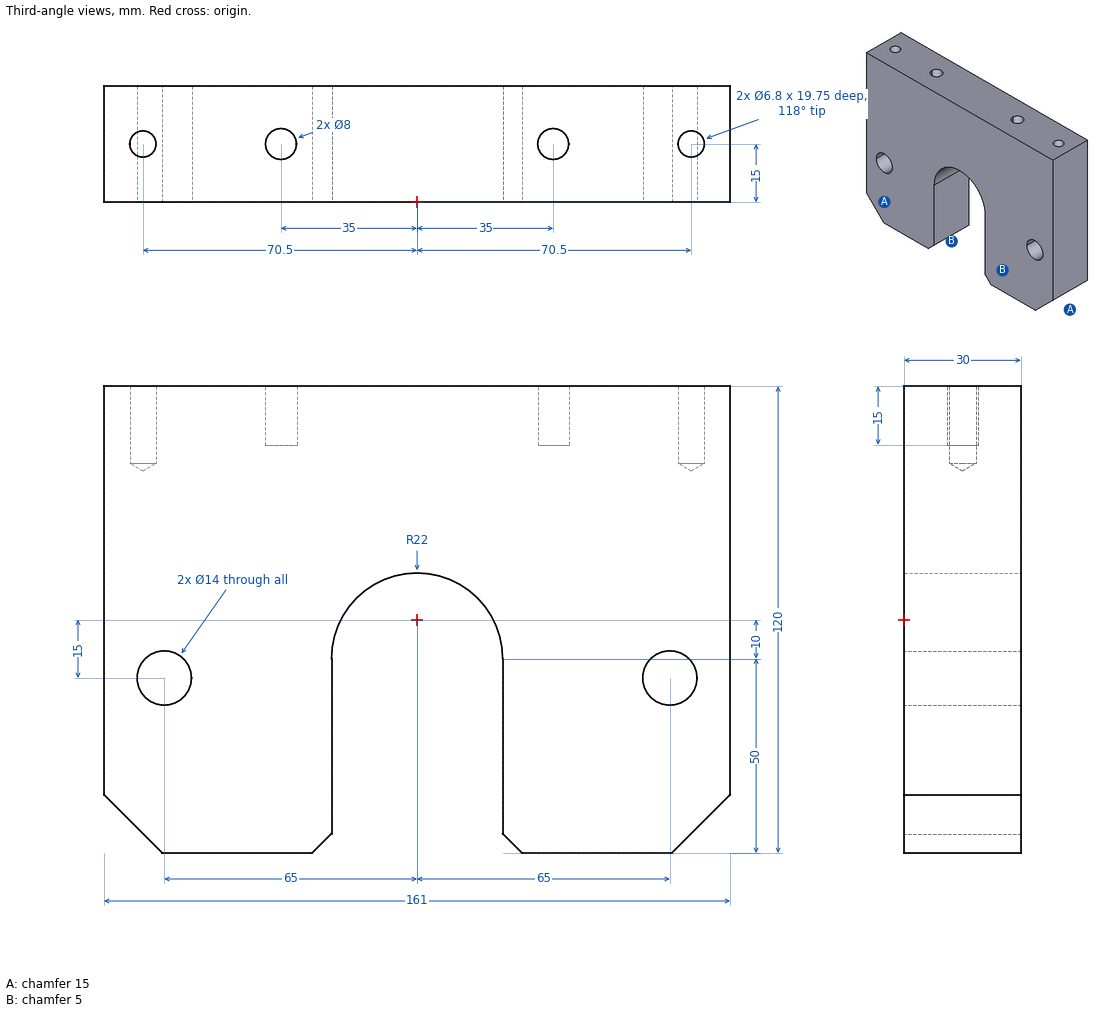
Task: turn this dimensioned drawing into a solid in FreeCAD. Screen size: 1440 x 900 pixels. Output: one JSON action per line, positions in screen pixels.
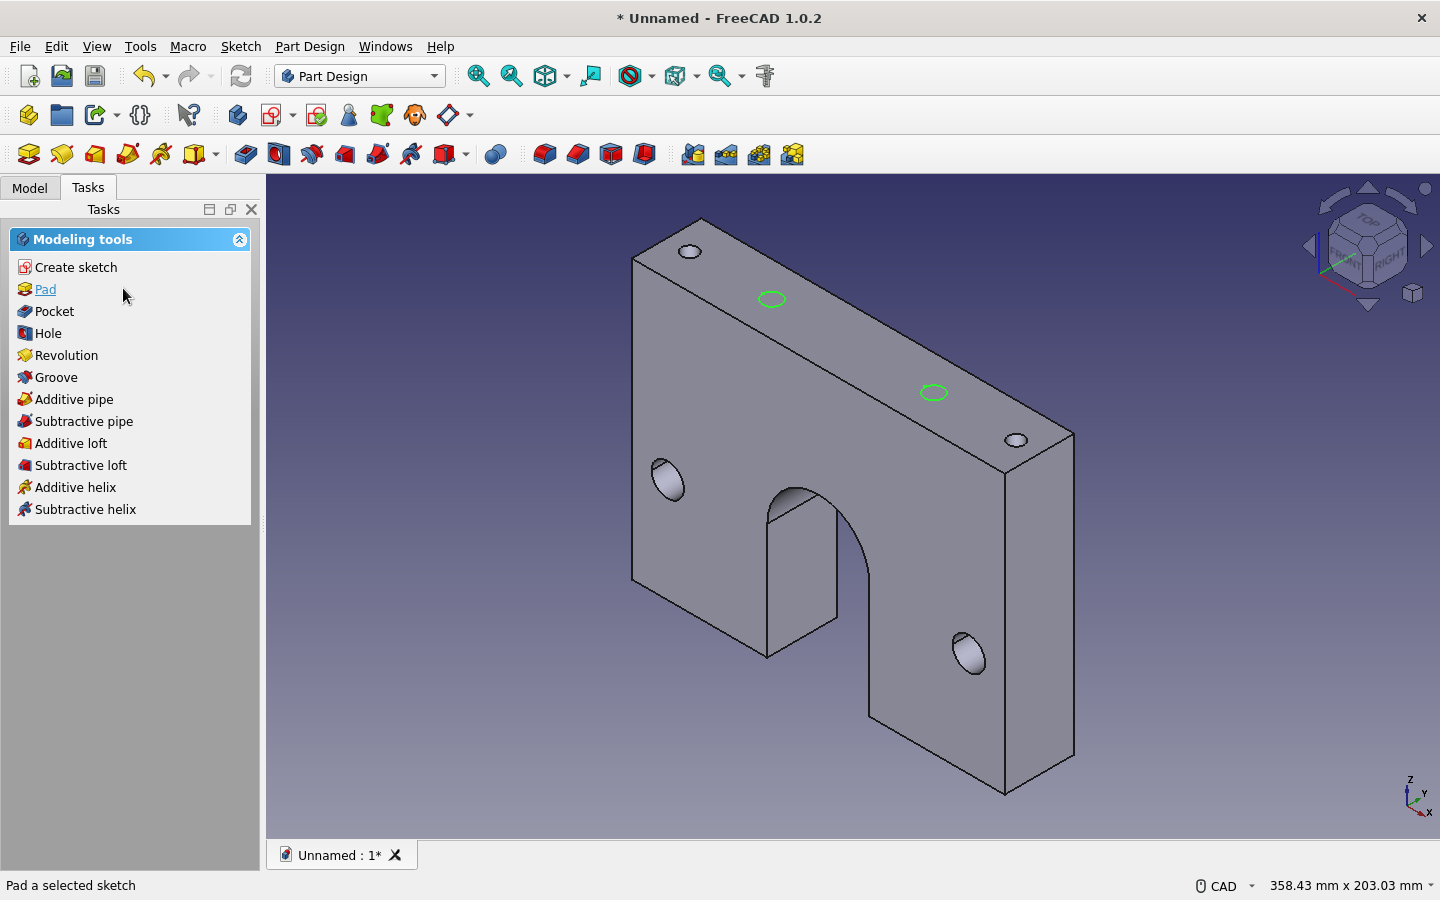
{"action": "left_click", "coordinate": [246, 154]}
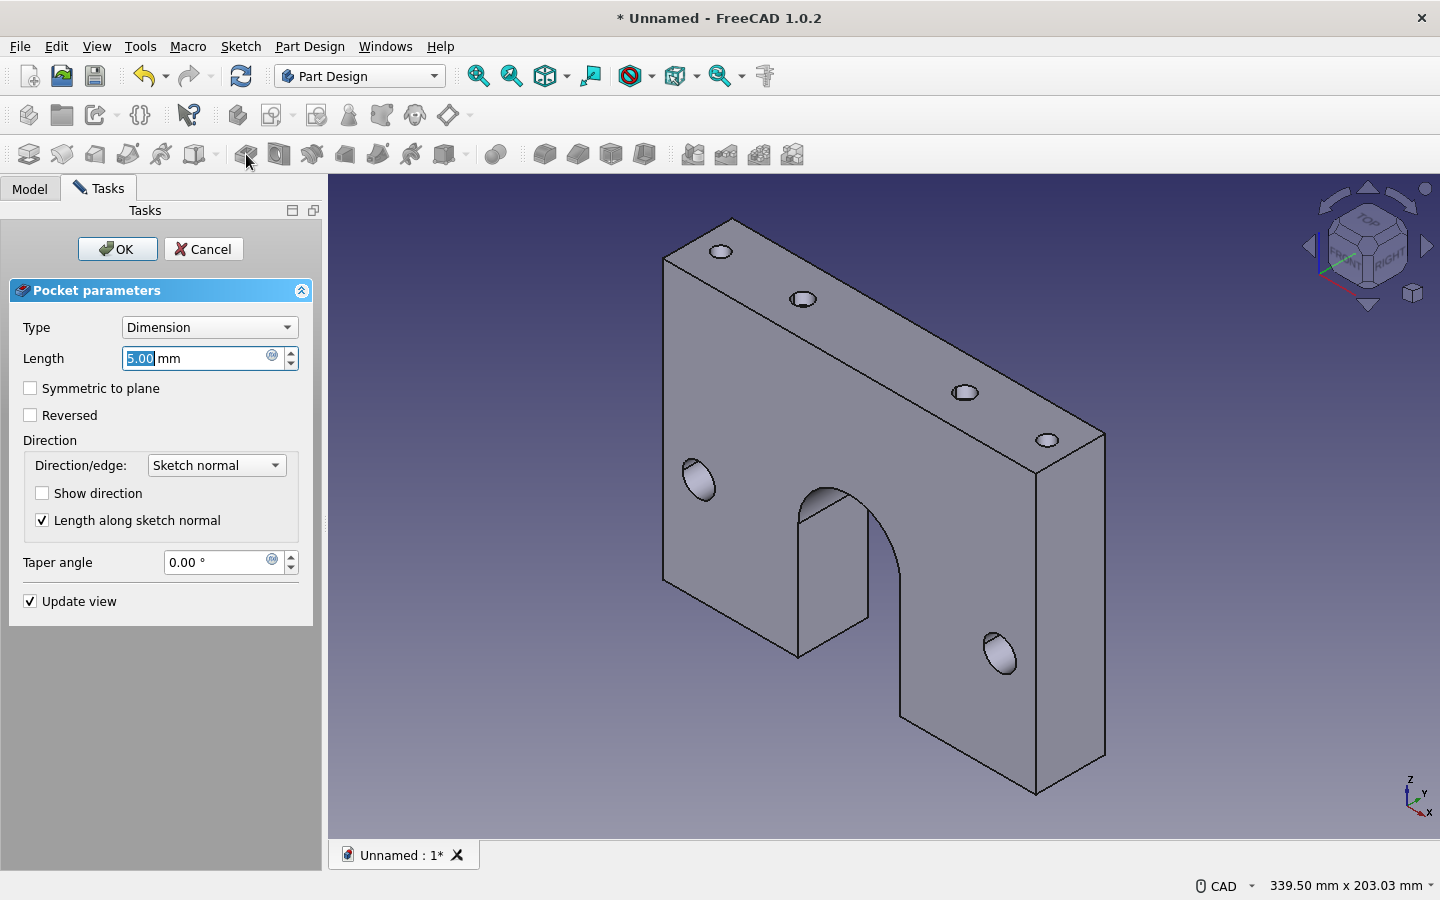
{"action": "type", "text": "15"}
{"action": "key", "text": "Tab"}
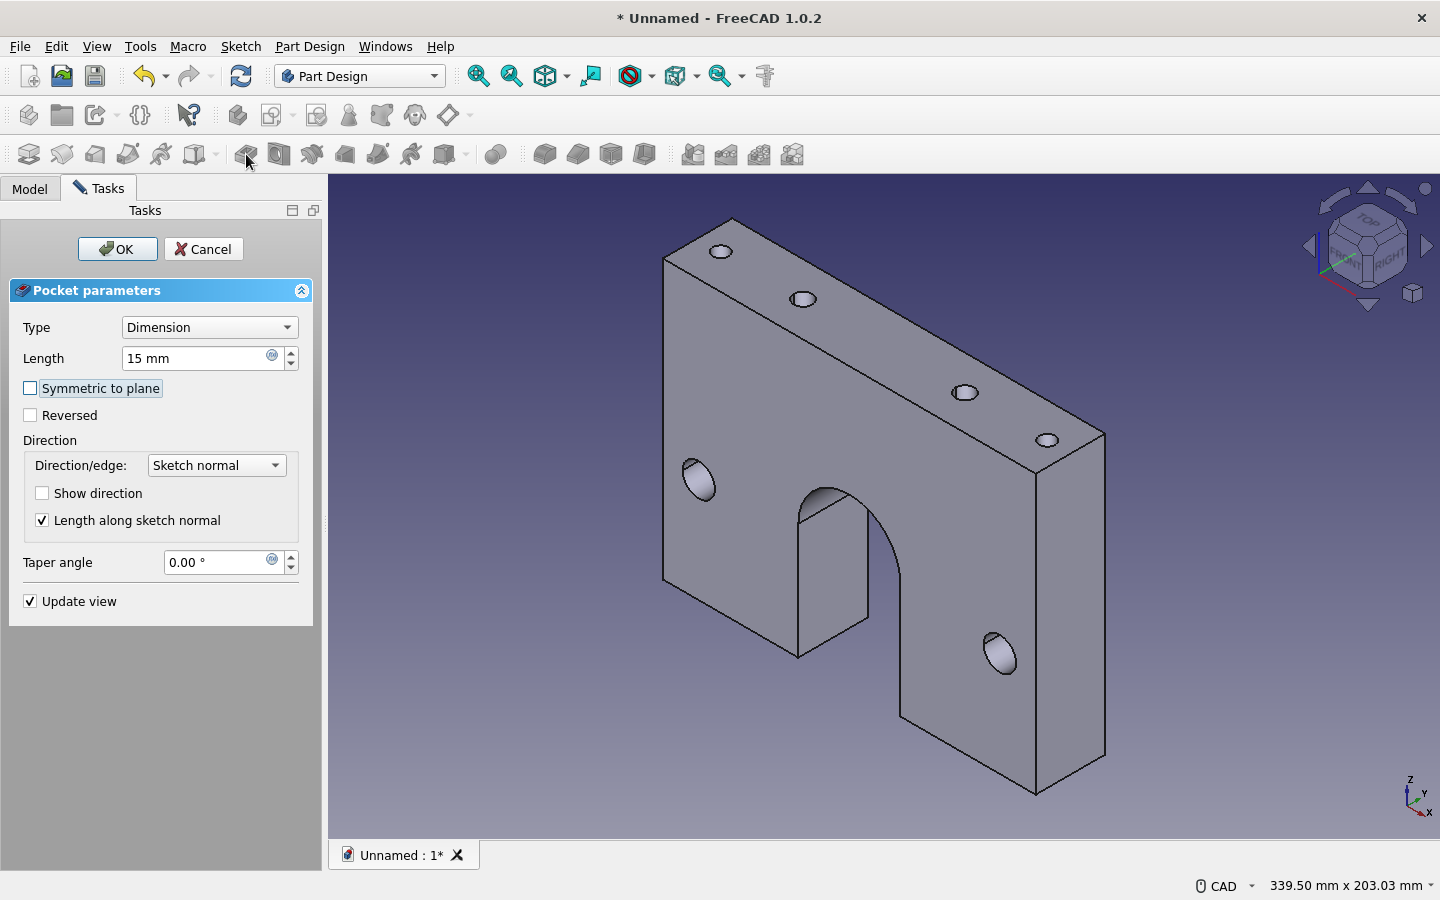
{"action": "left_click", "coordinate": [118, 249]}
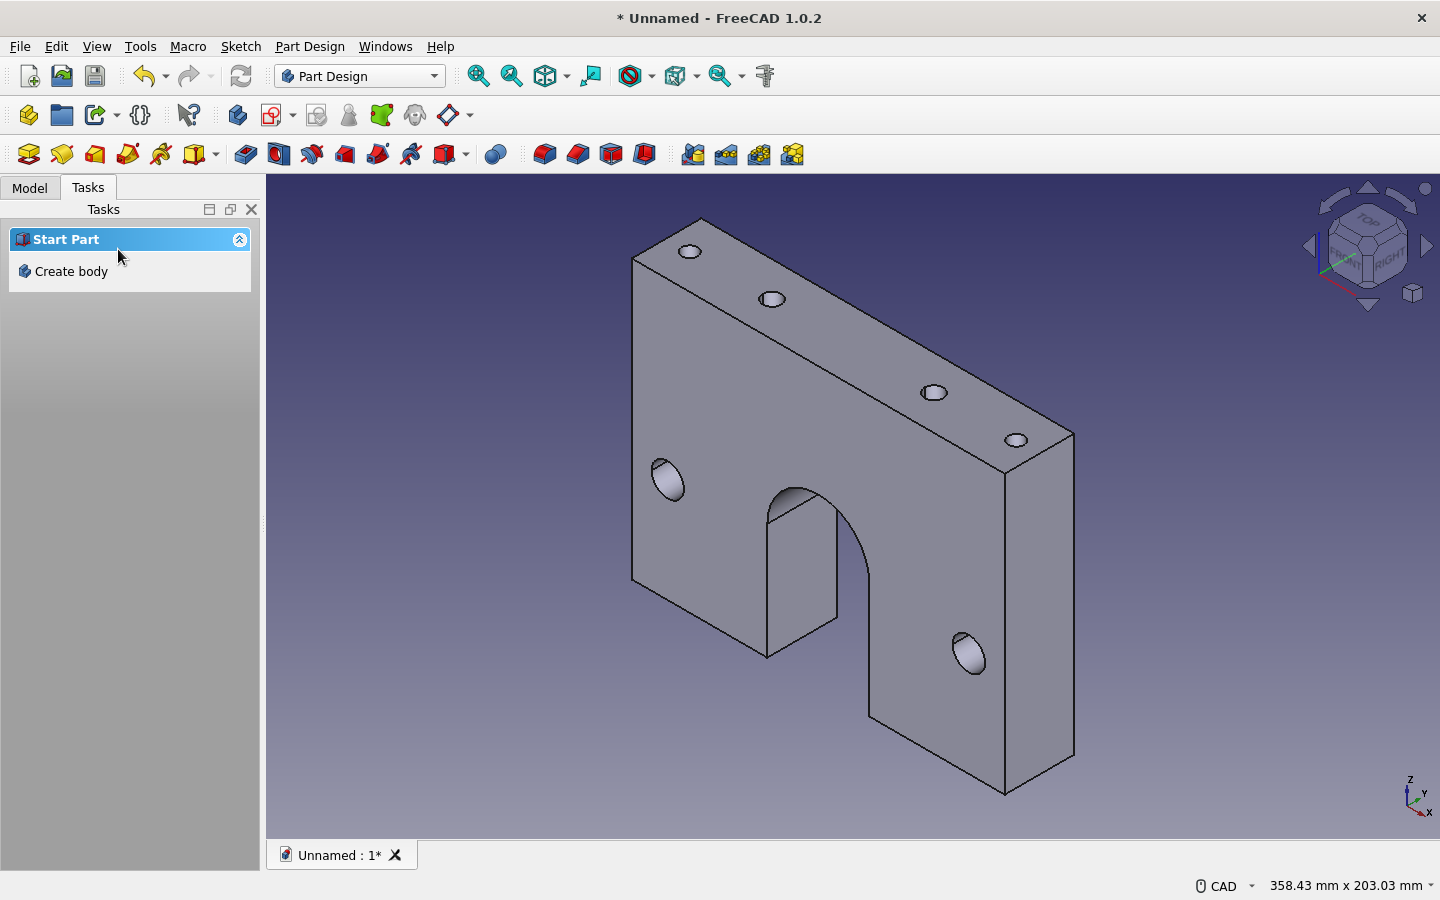
{"action": "key", "text": "2"}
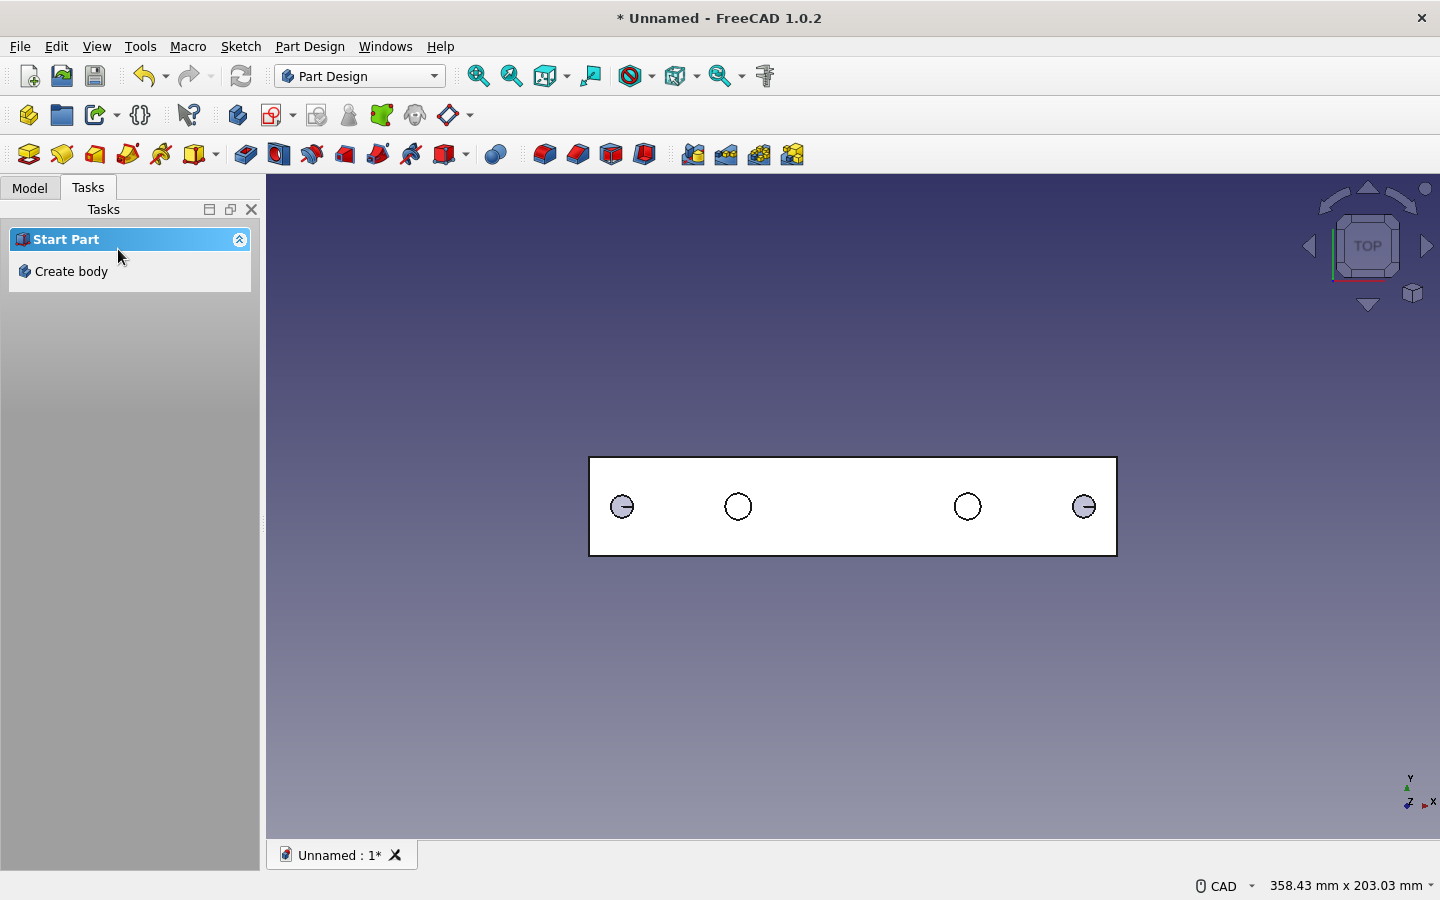
{"action": "key", "text": "v f"}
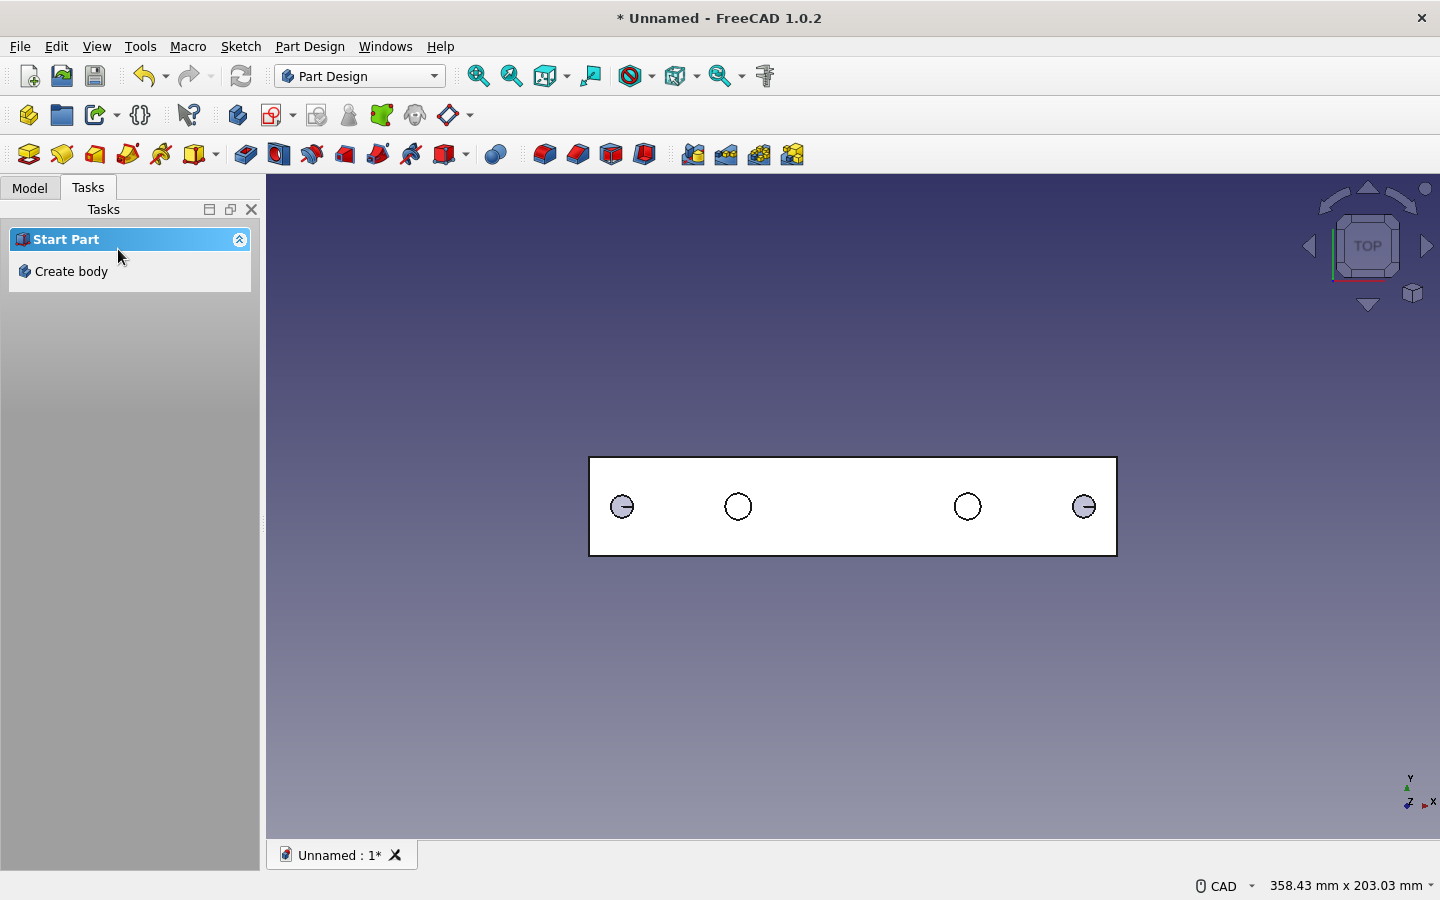
{"action": "key", "text": "0"}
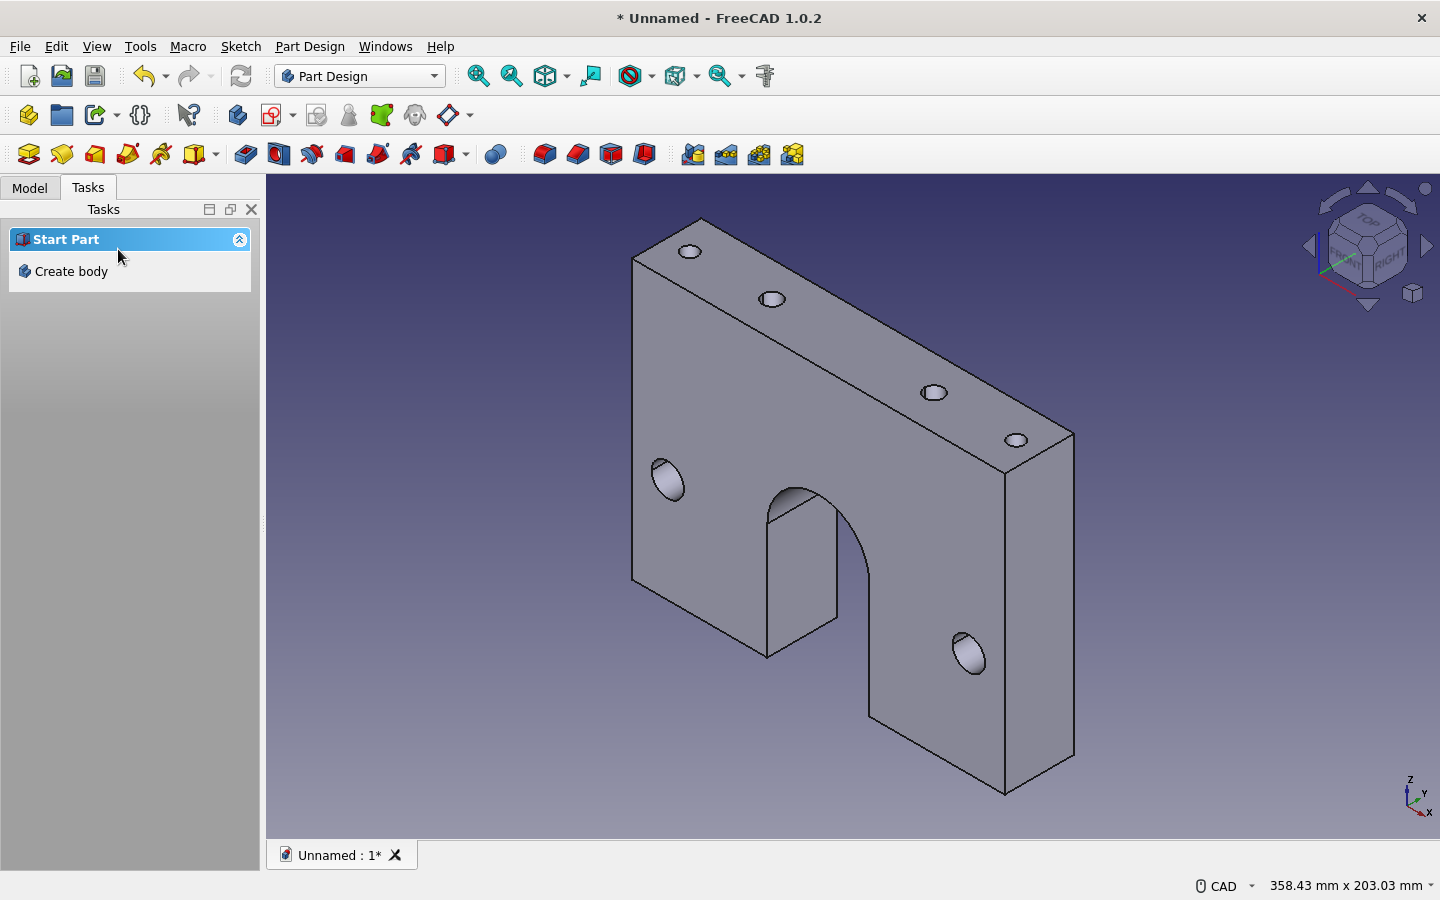
{"action": "key", "text": "1"}